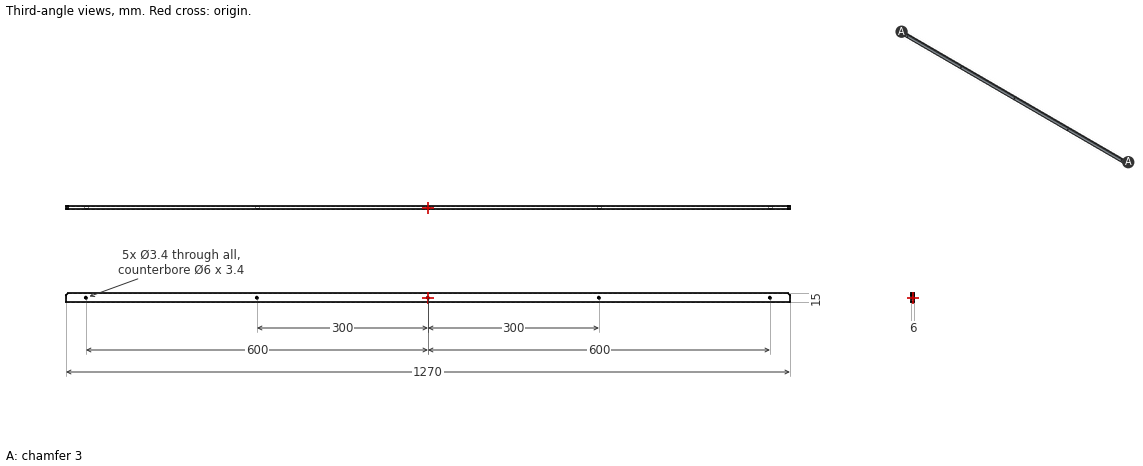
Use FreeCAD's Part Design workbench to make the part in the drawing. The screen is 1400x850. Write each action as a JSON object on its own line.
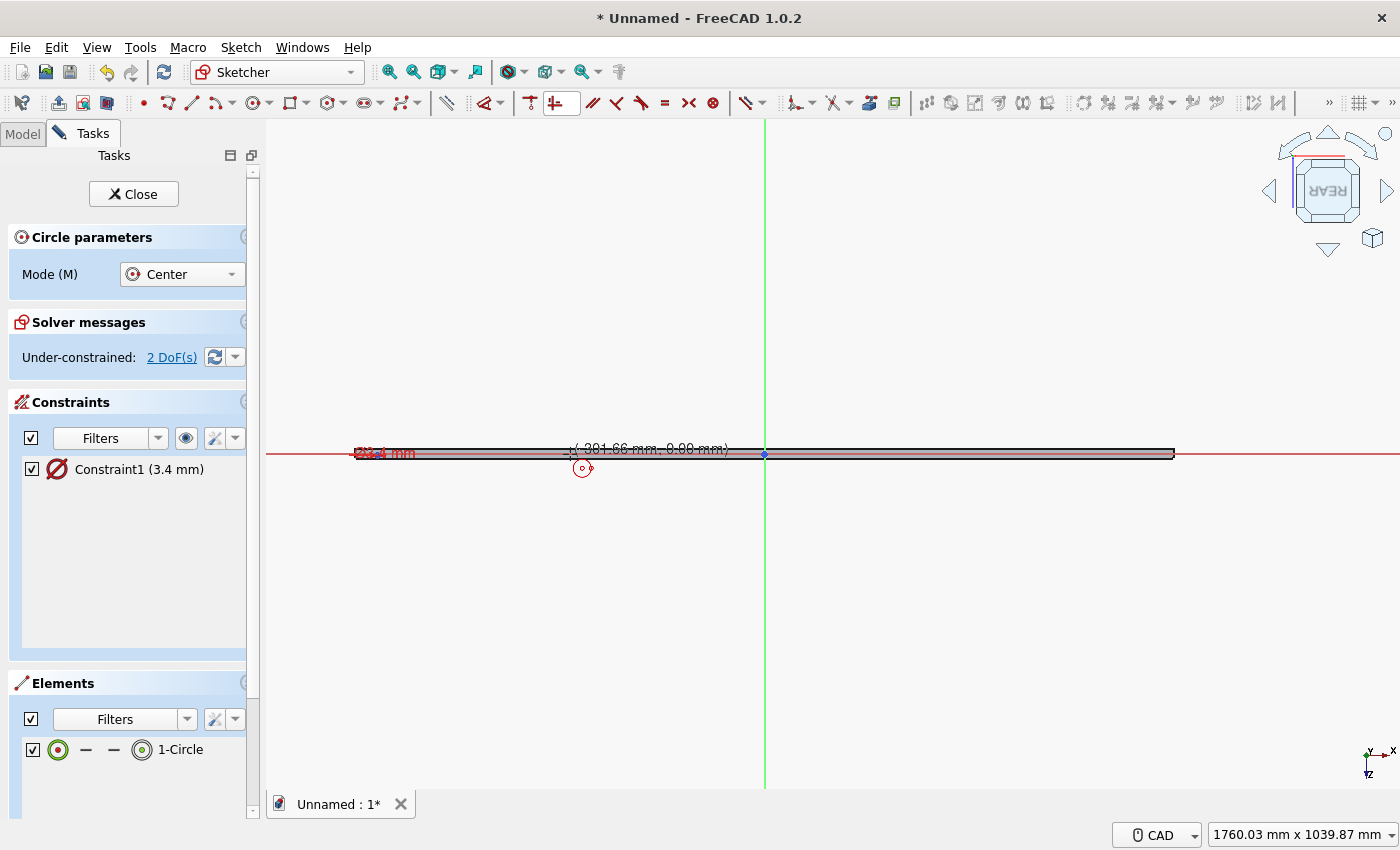
{"action": "left_click", "coordinate": [571, 454]}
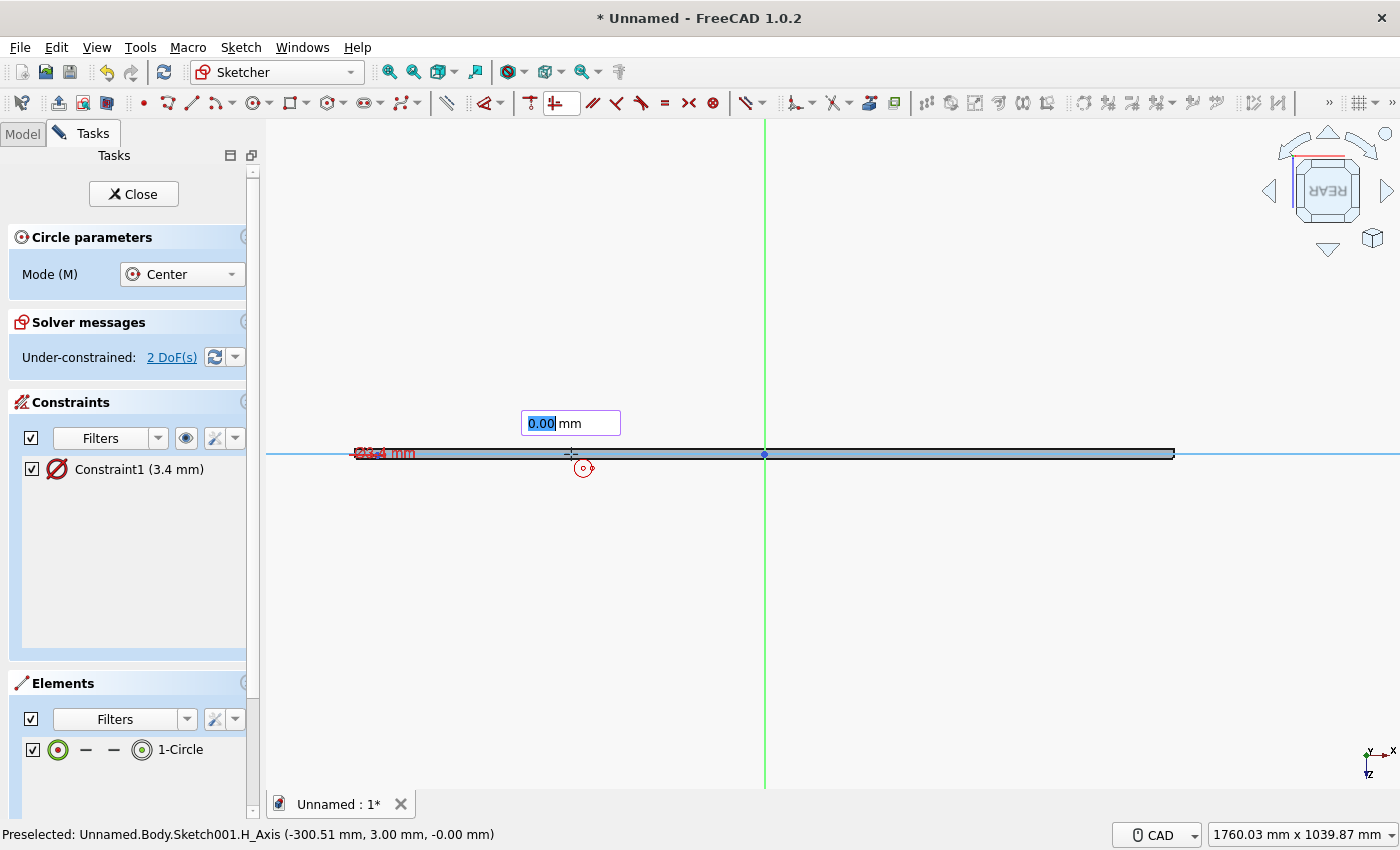
{"action": "scroll", "coordinate": [572, 453], "scroll_direction": "up", "scroll_amount": 14}
{"action": "mouse_move", "coordinate": [563, 447]}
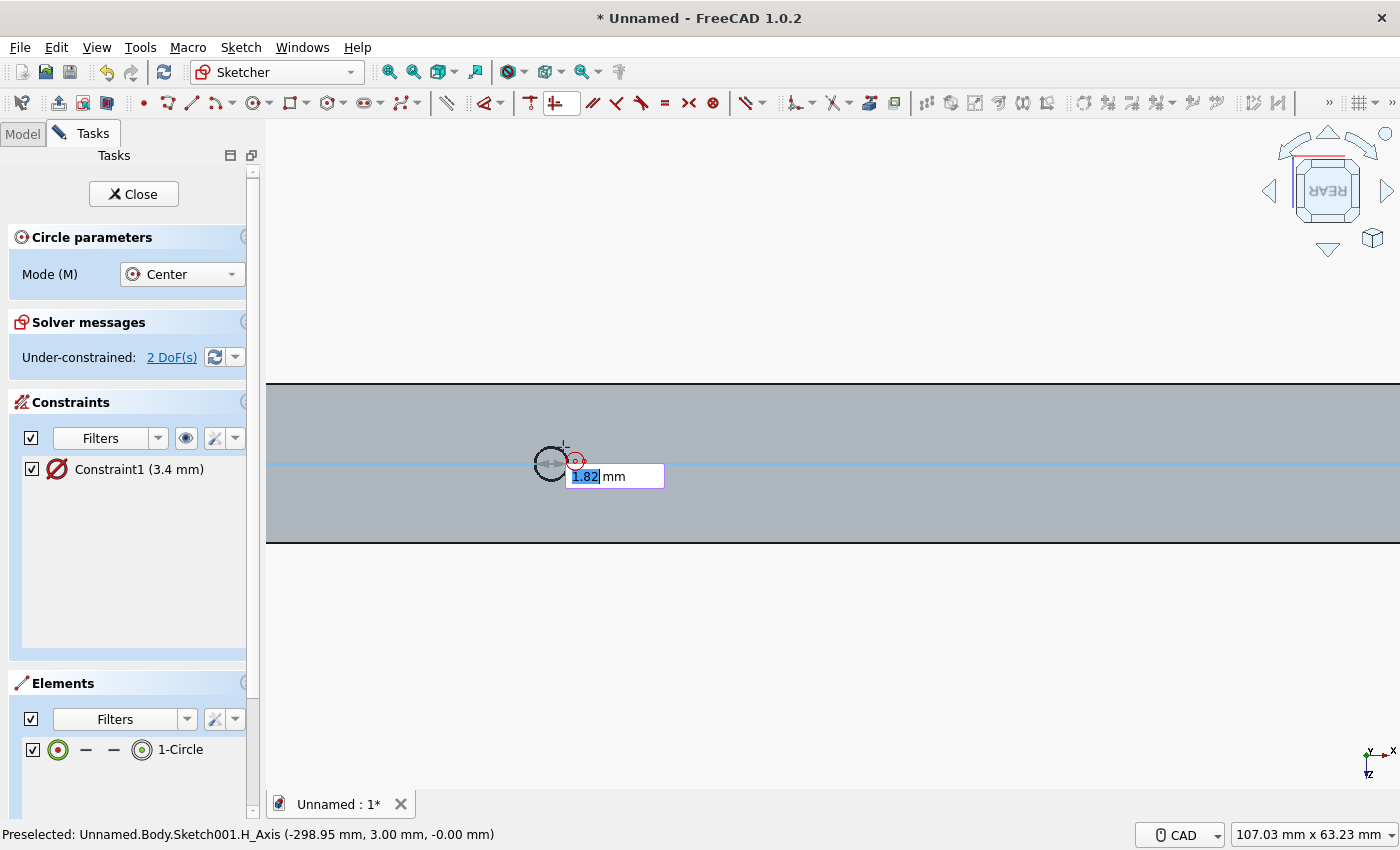
{"action": "type", "text": "3.4"}
{"action": "key", "text": "Return"}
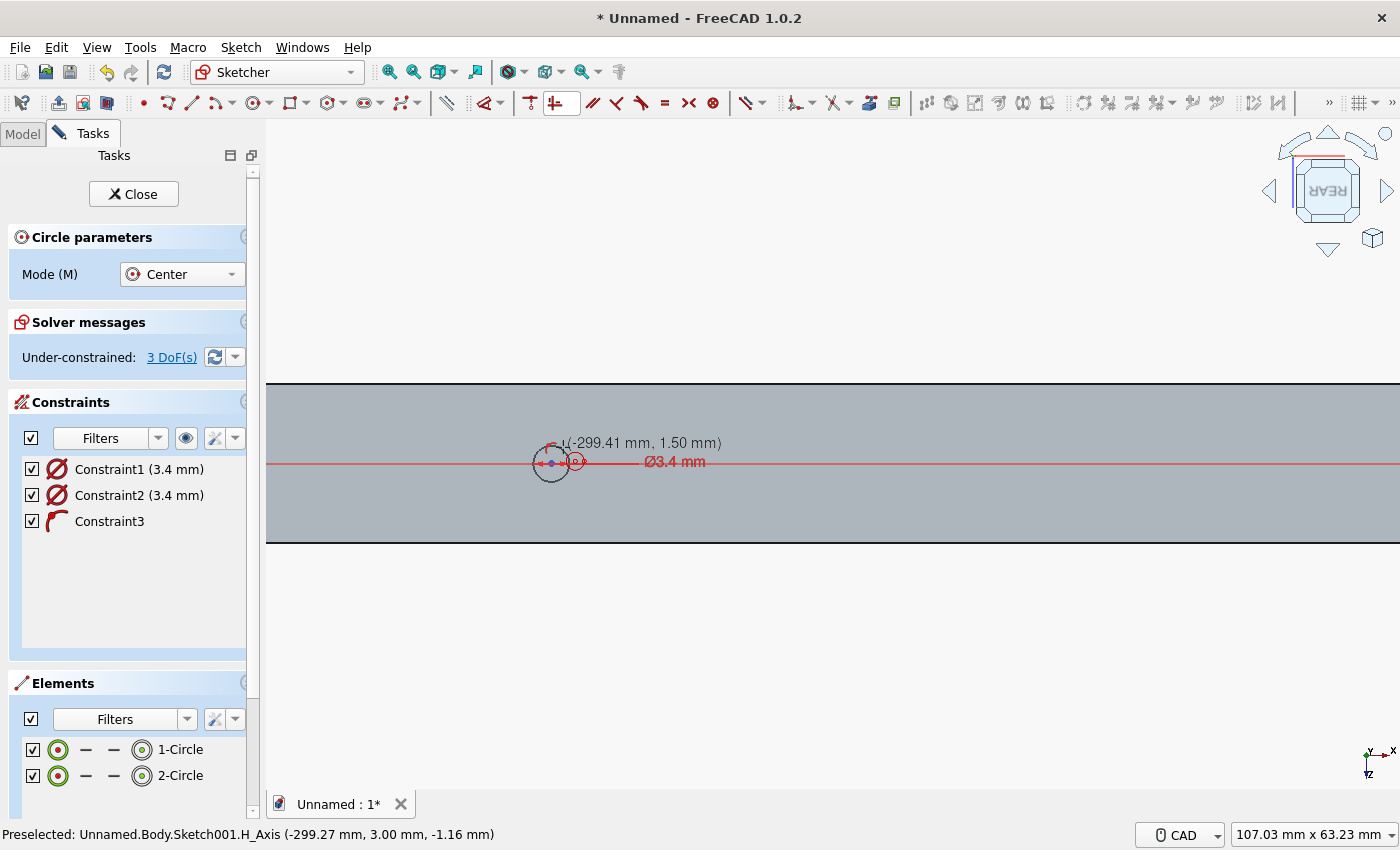
{"action": "scroll", "coordinate": [609, 453], "scroll_direction": "down", "scroll_amount": 15}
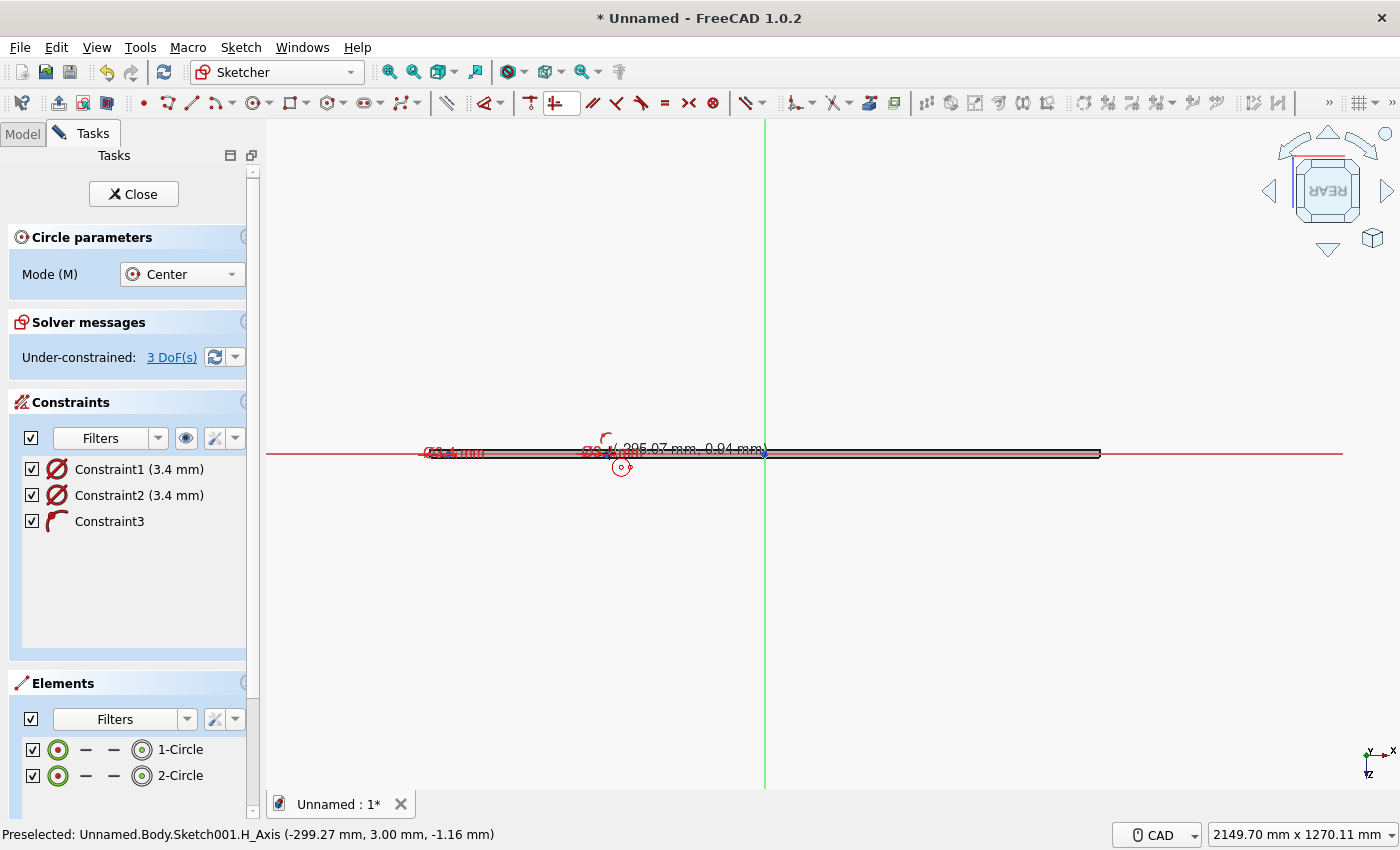
{"action": "scroll", "coordinate": [765, 454], "scroll_direction": "up", "scroll_amount": 17}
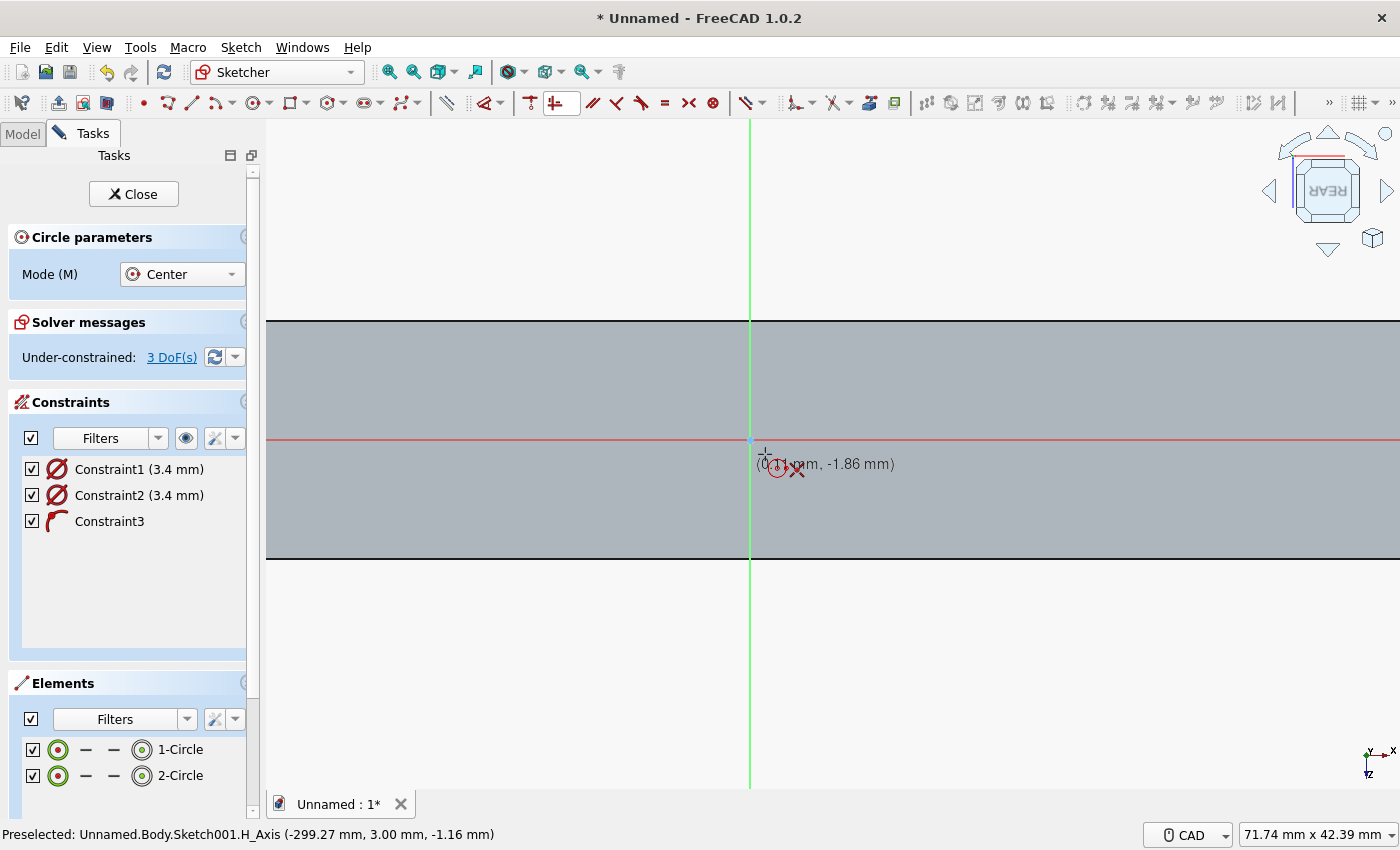
{"action": "scroll", "coordinate": [765, 455], "scroll_direction": "down", "scroll_amount": 16}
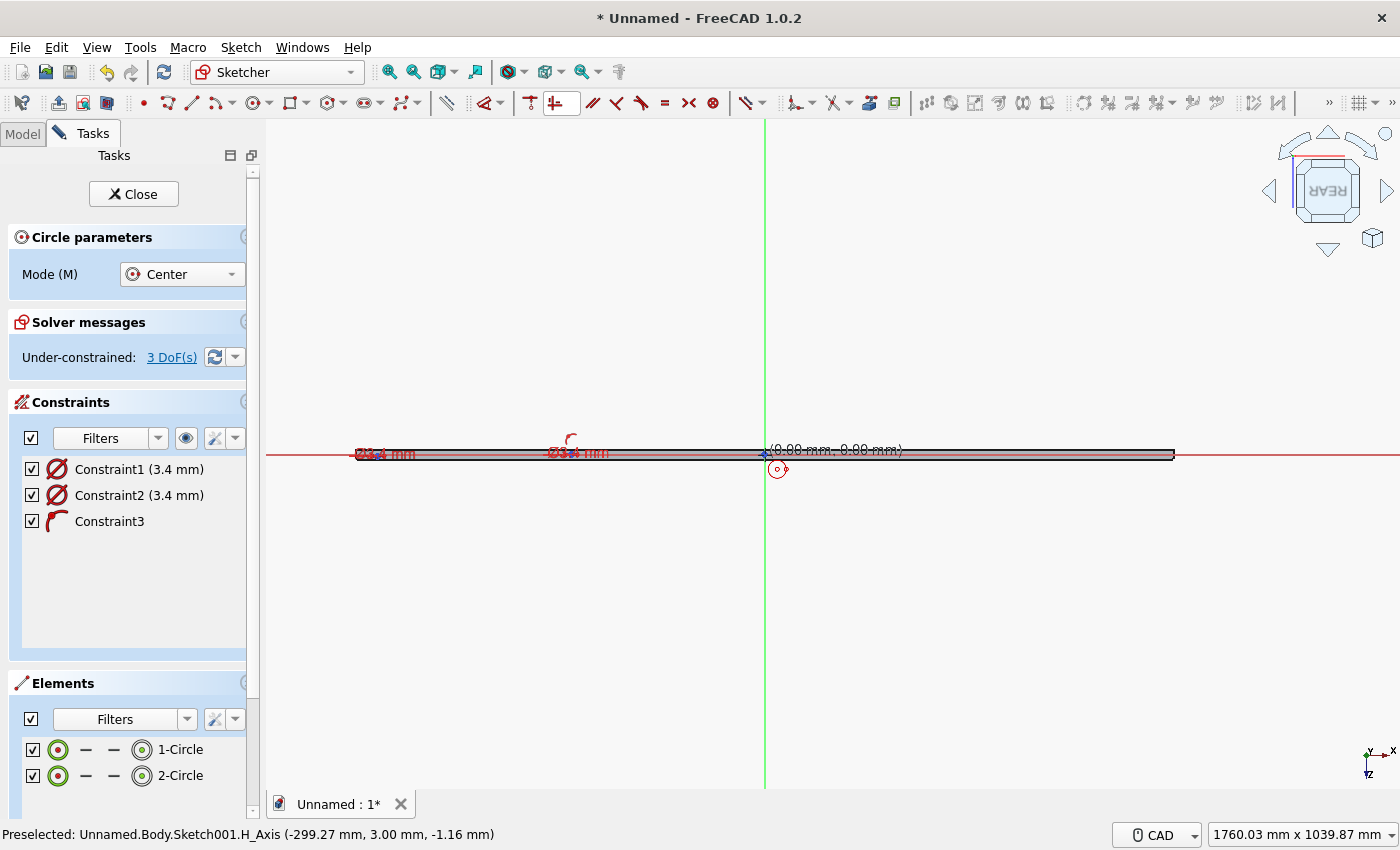
{"action": "left_click", "coordinate": [765, 455]}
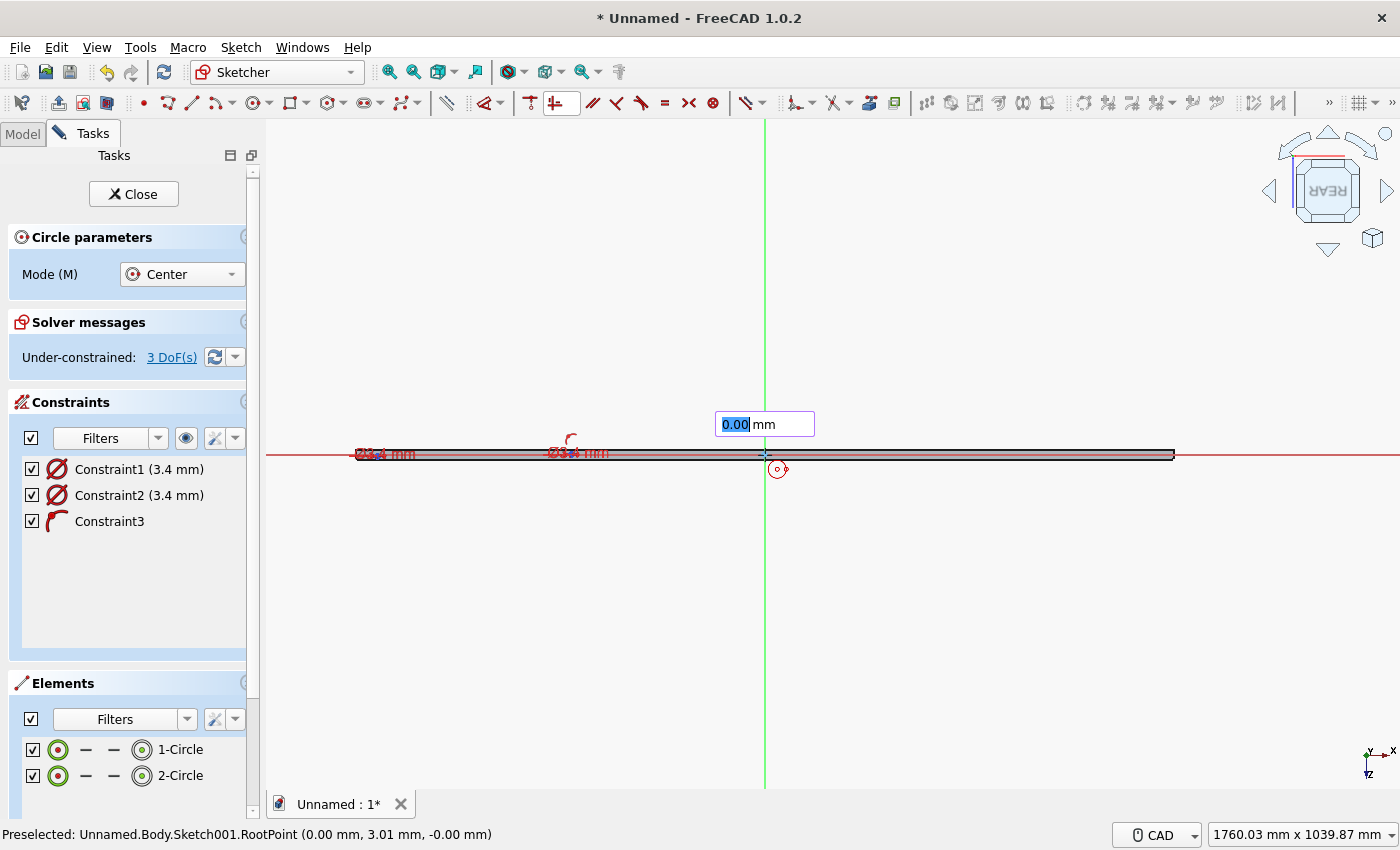
{"action": "scroll", "coordinate": [766, 454], "scroll_direction": "up", "scroll_amount": 16}
{"action": "mouse_move", "coordinate": [746, 445]}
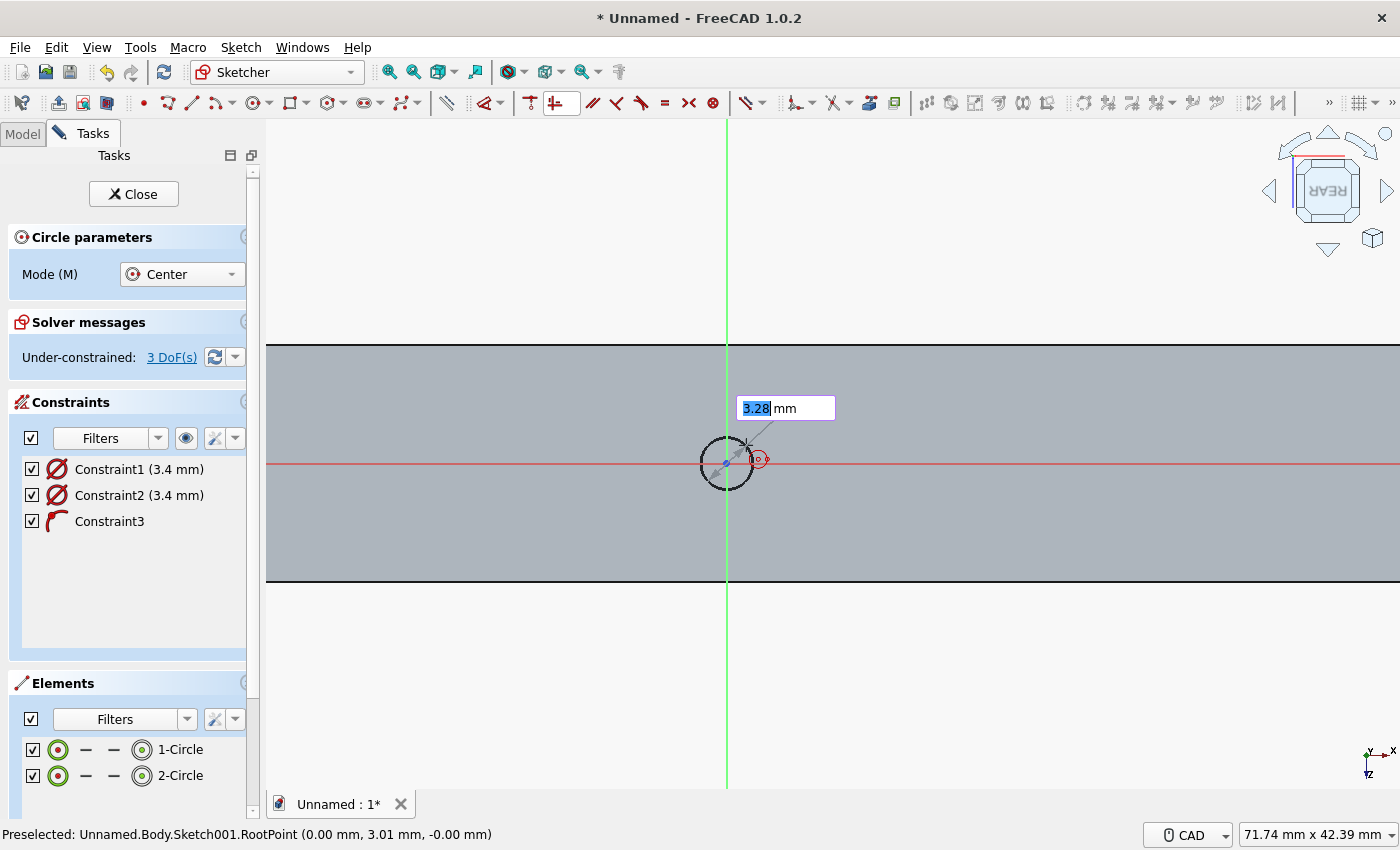
{"action": "type", "text": "3.4"}
{"action": "key", "text": "Return"}